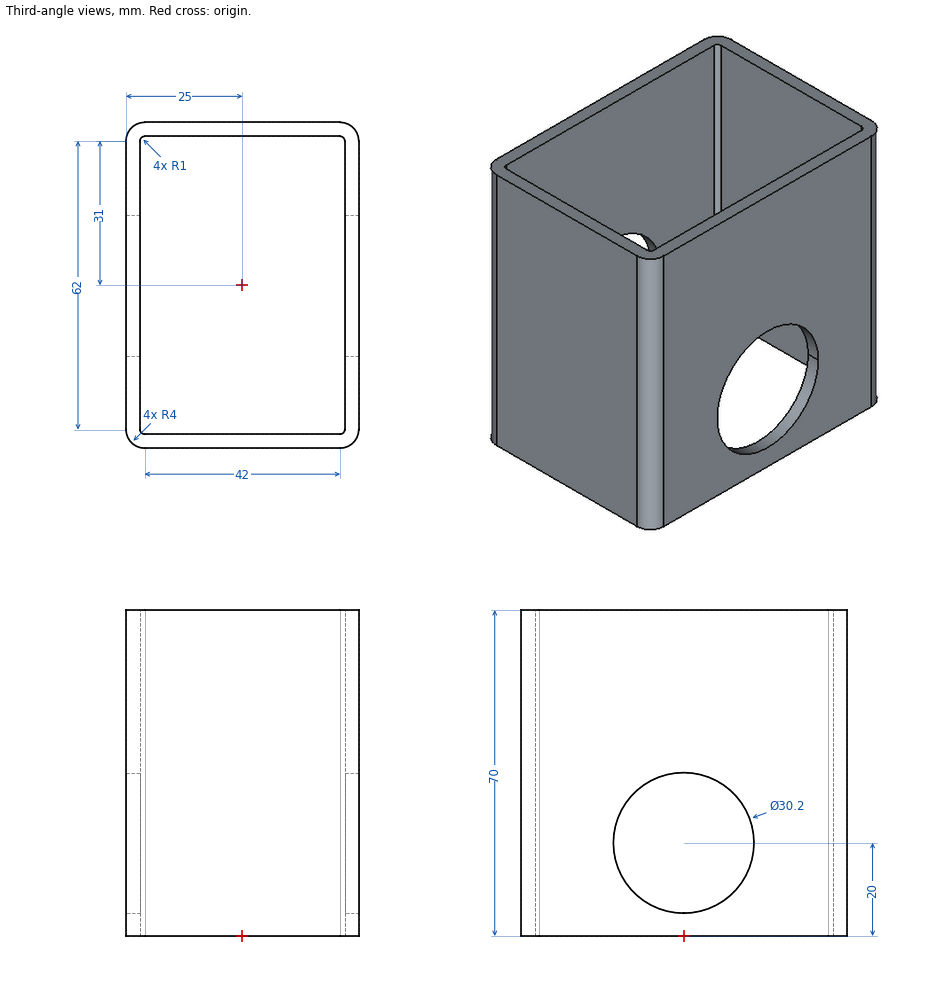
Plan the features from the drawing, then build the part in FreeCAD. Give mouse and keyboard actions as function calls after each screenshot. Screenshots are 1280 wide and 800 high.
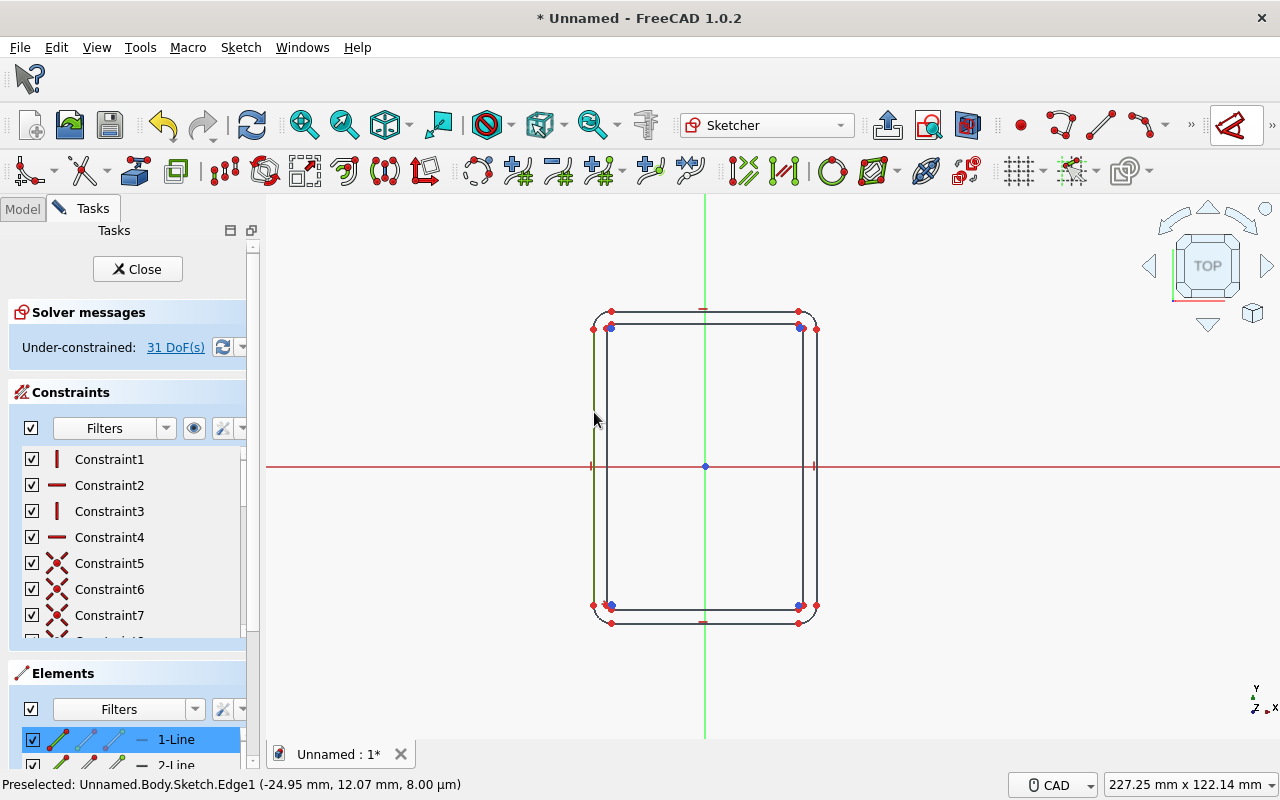
click(599, 317)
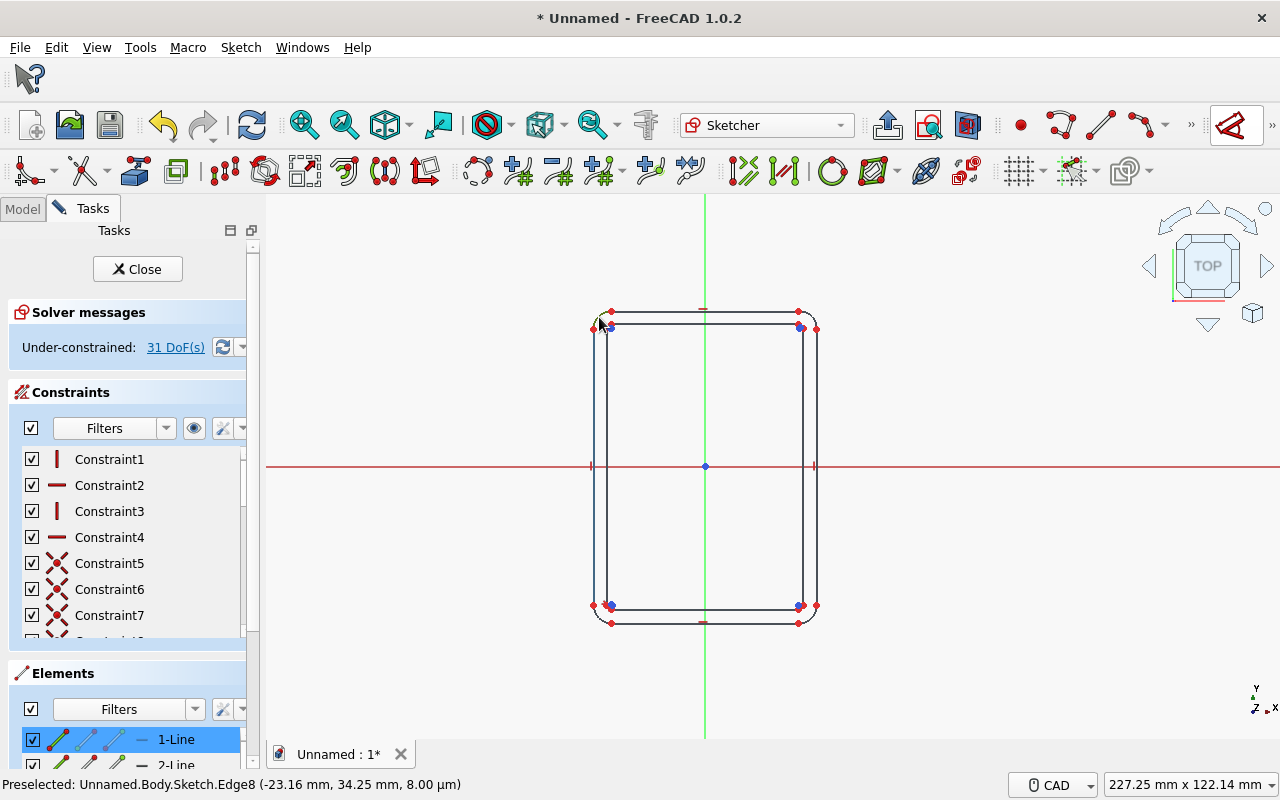
key(t)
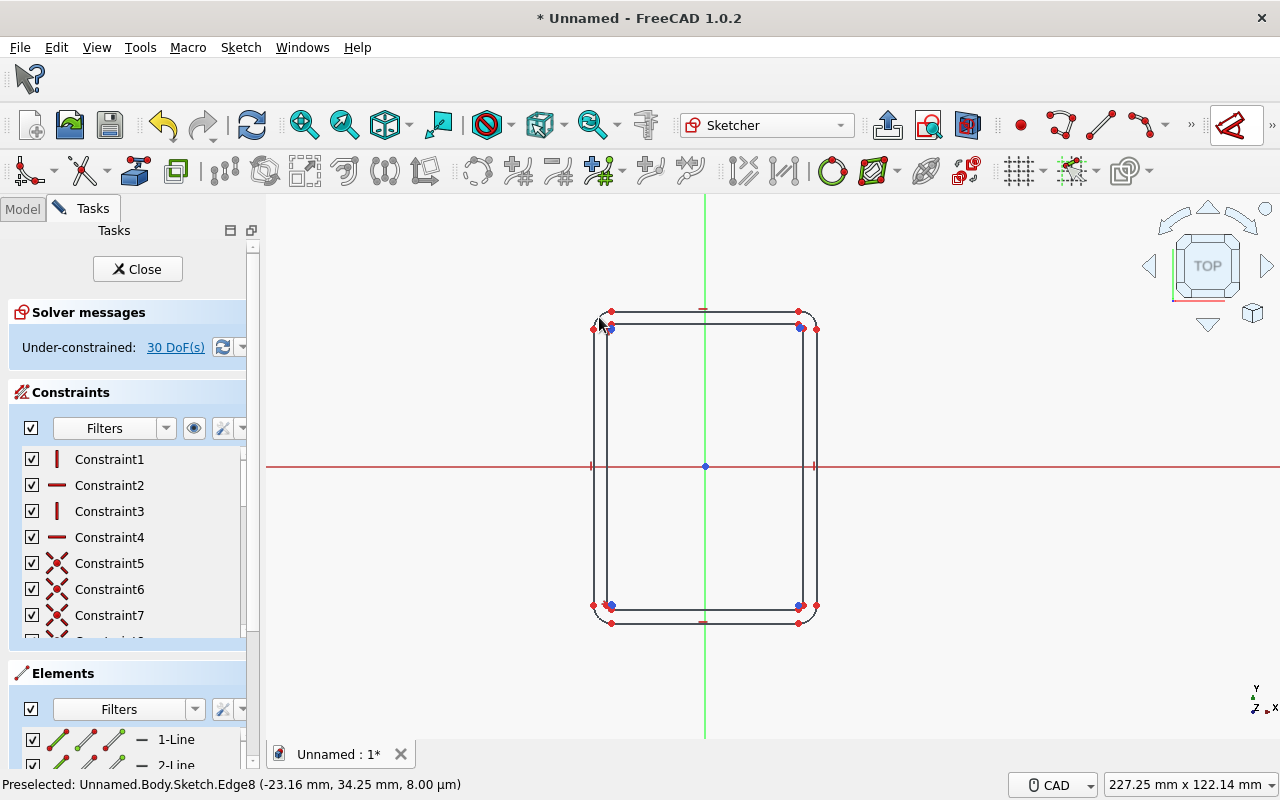
click(668, 624)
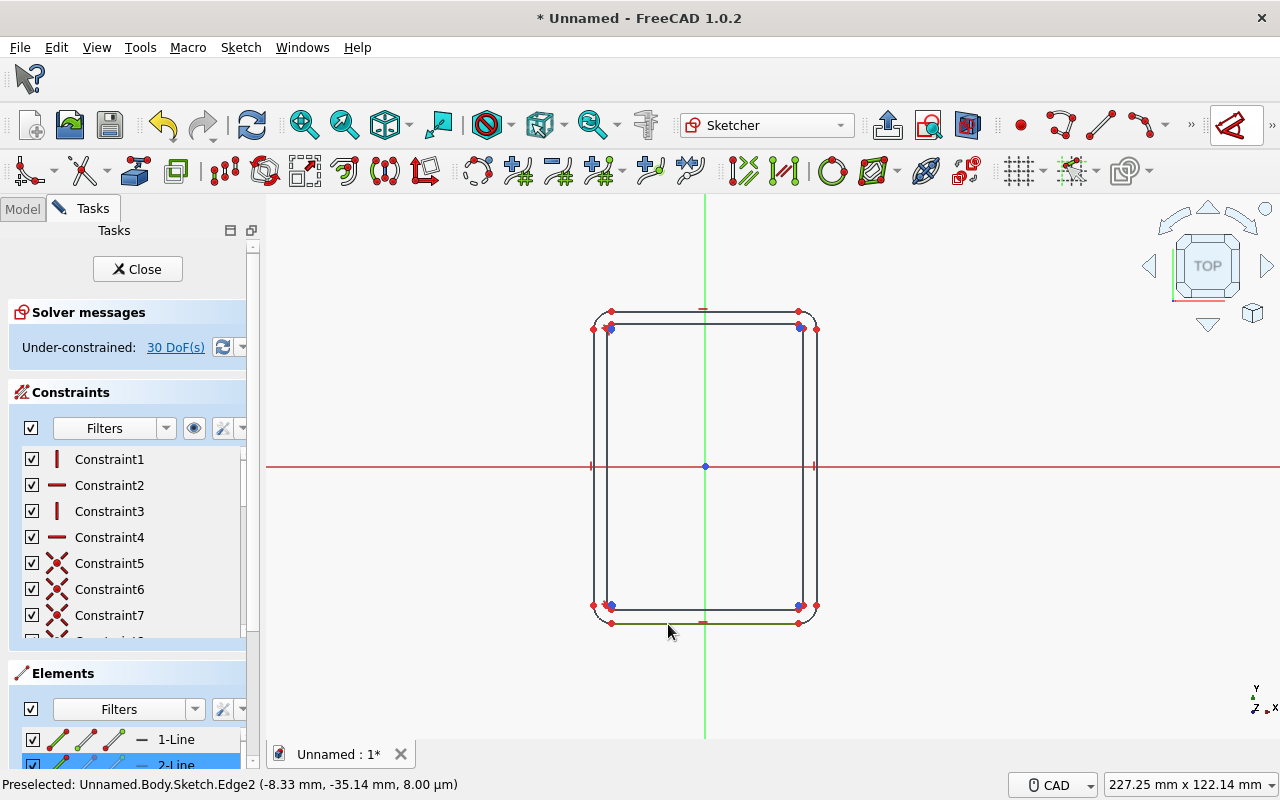
click(599, 618)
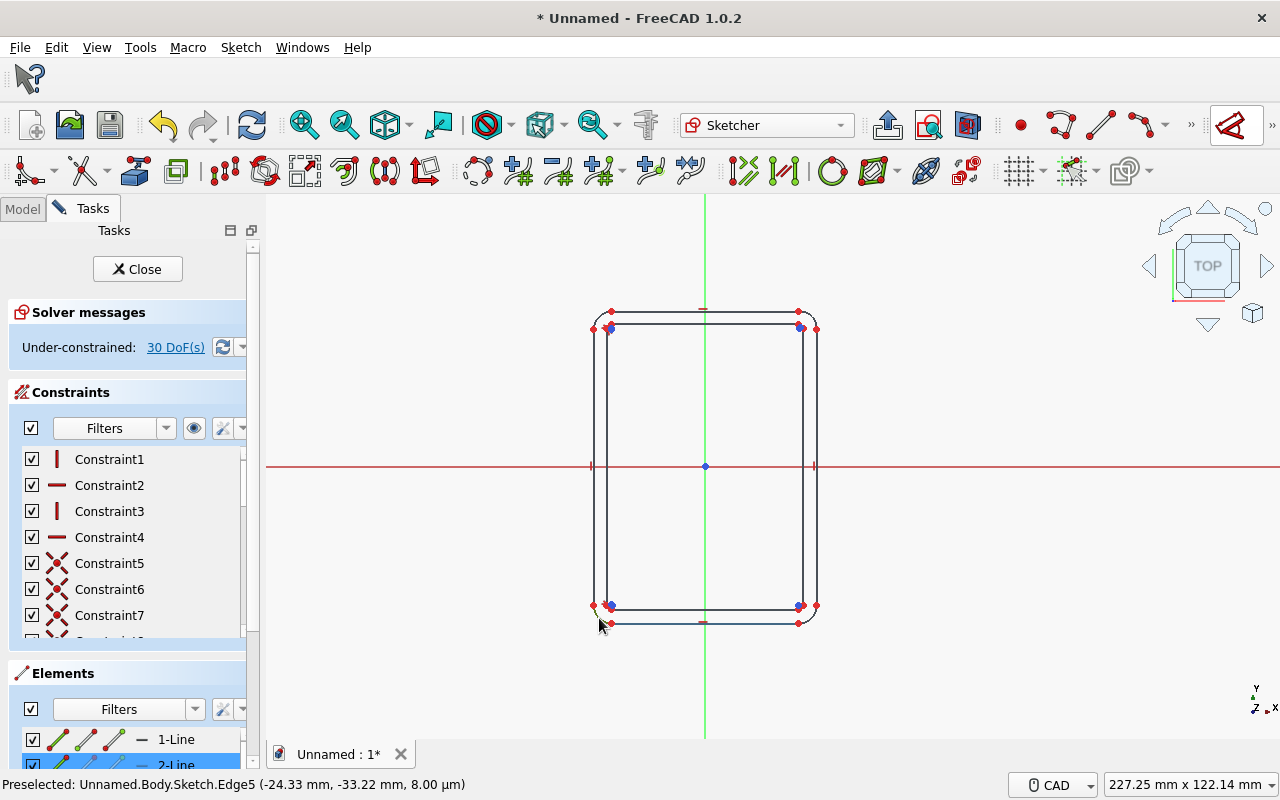
key(t)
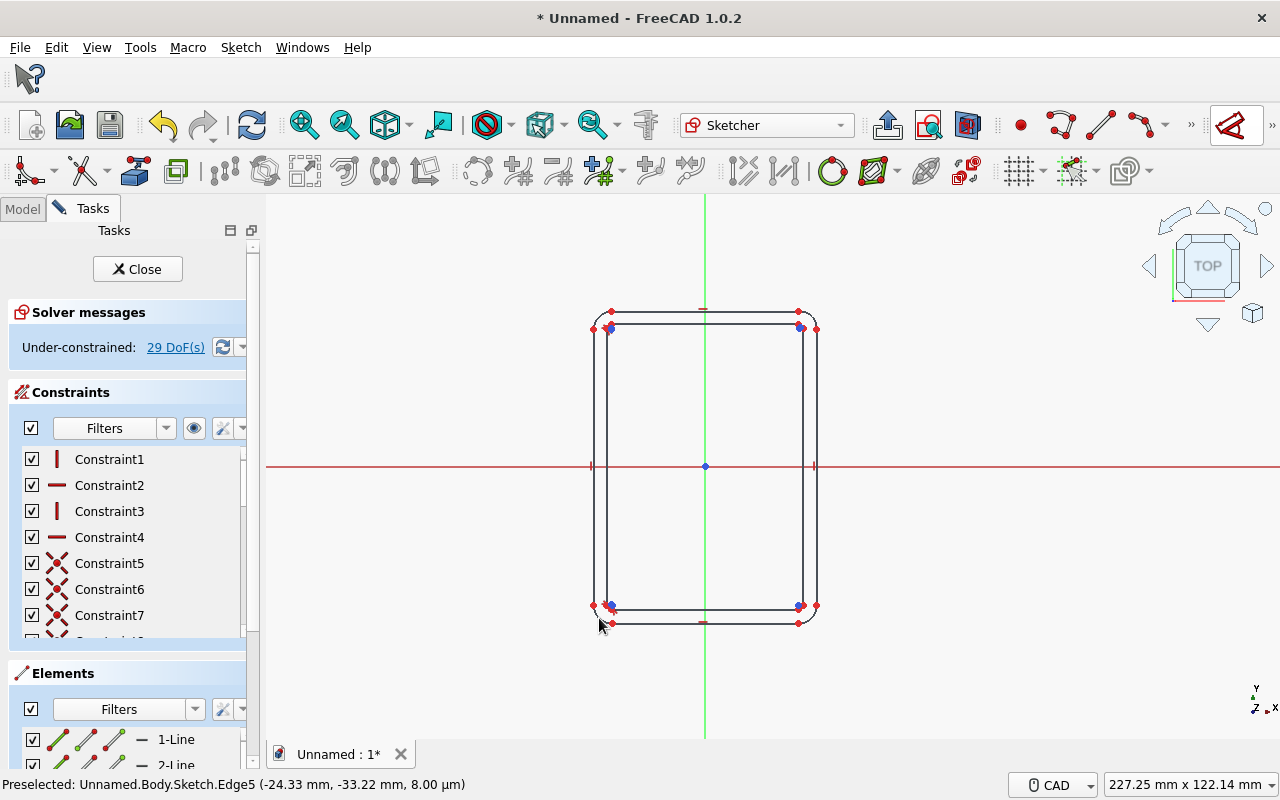
click(668, 624)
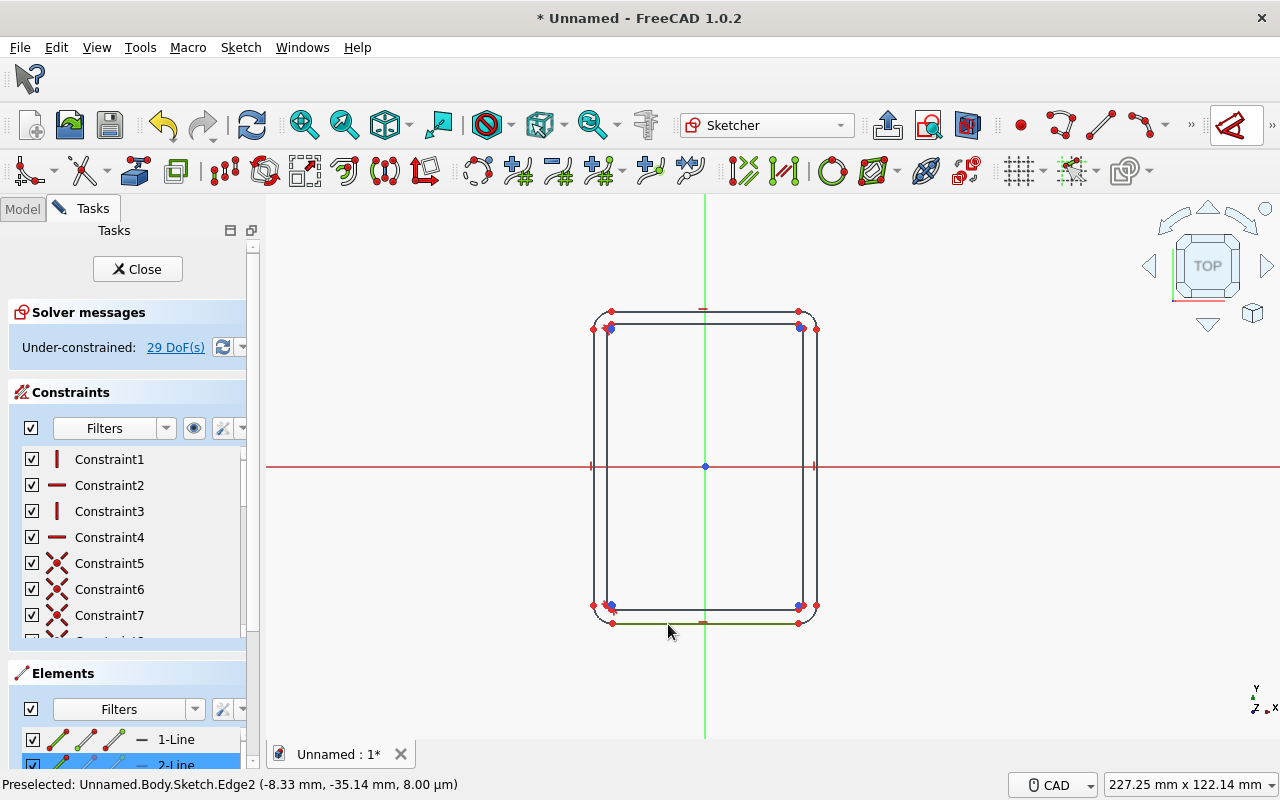
click(811, 618)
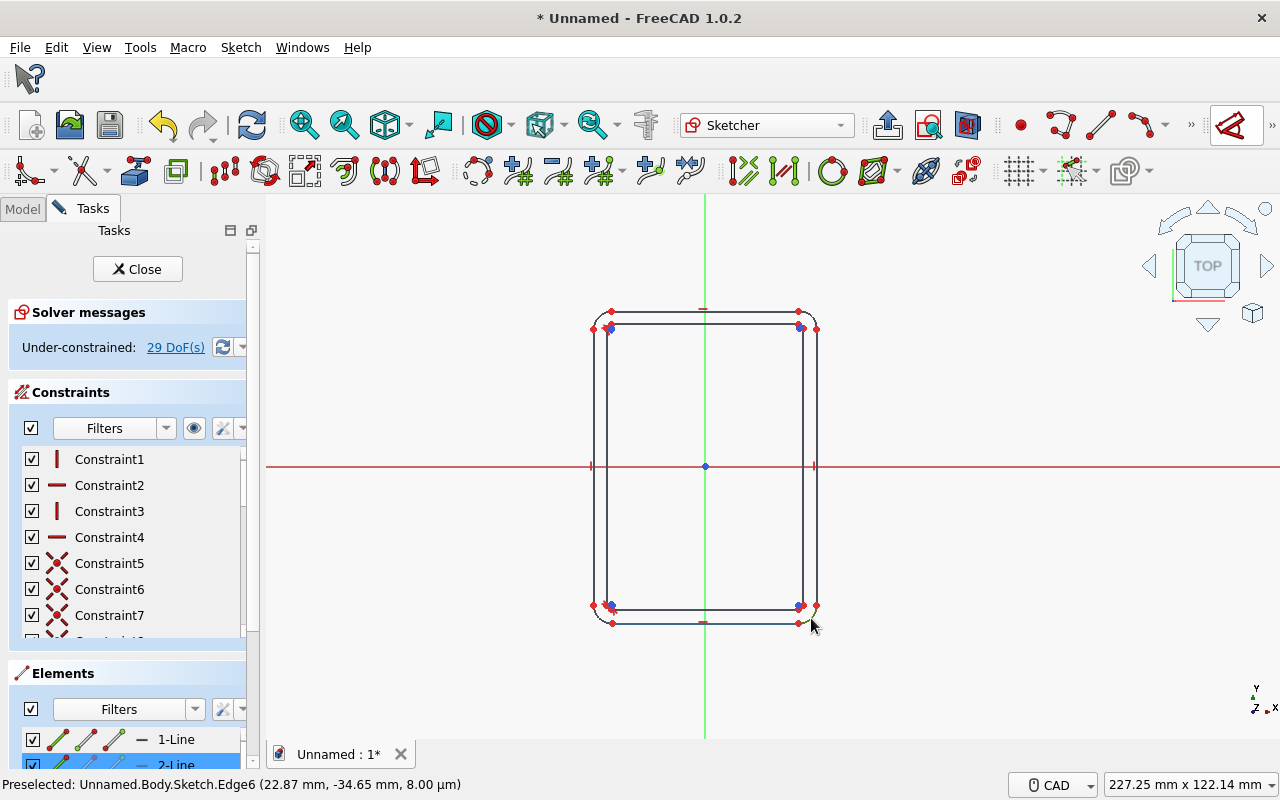
key(t)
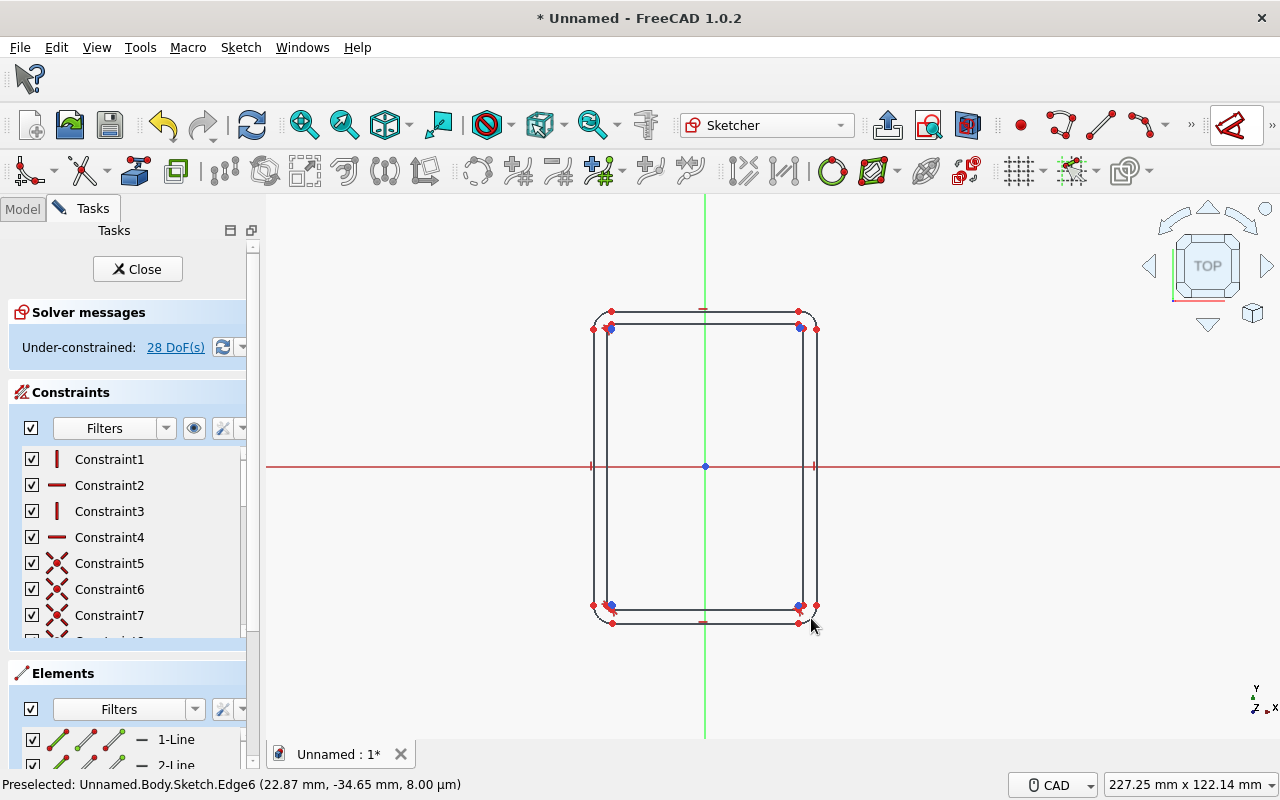
click(817, 523)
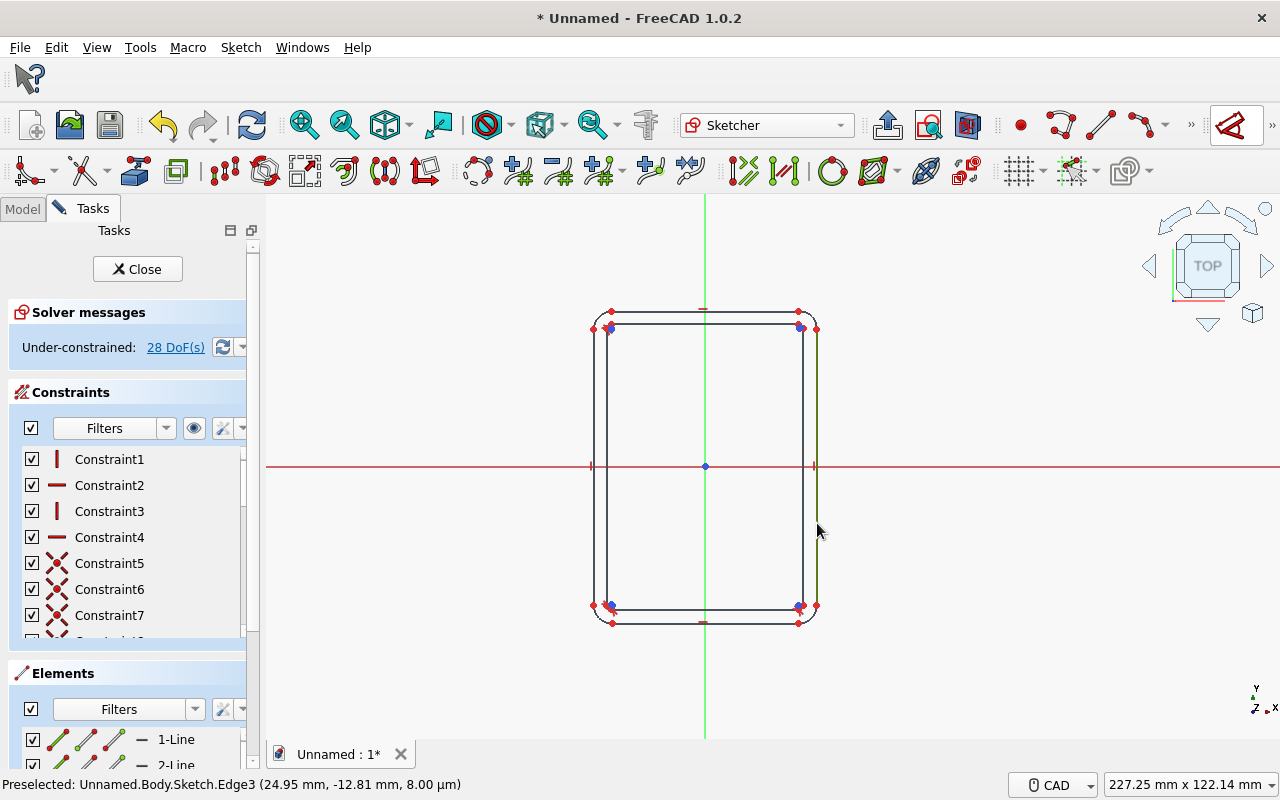
click(811, 618)